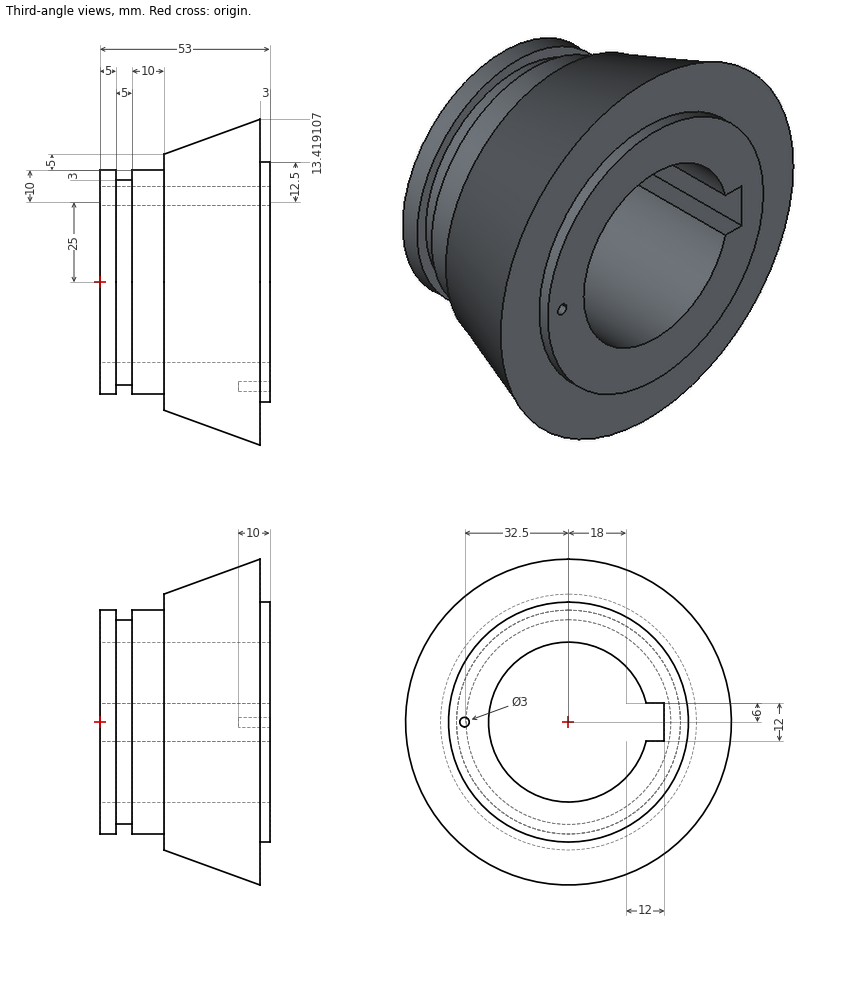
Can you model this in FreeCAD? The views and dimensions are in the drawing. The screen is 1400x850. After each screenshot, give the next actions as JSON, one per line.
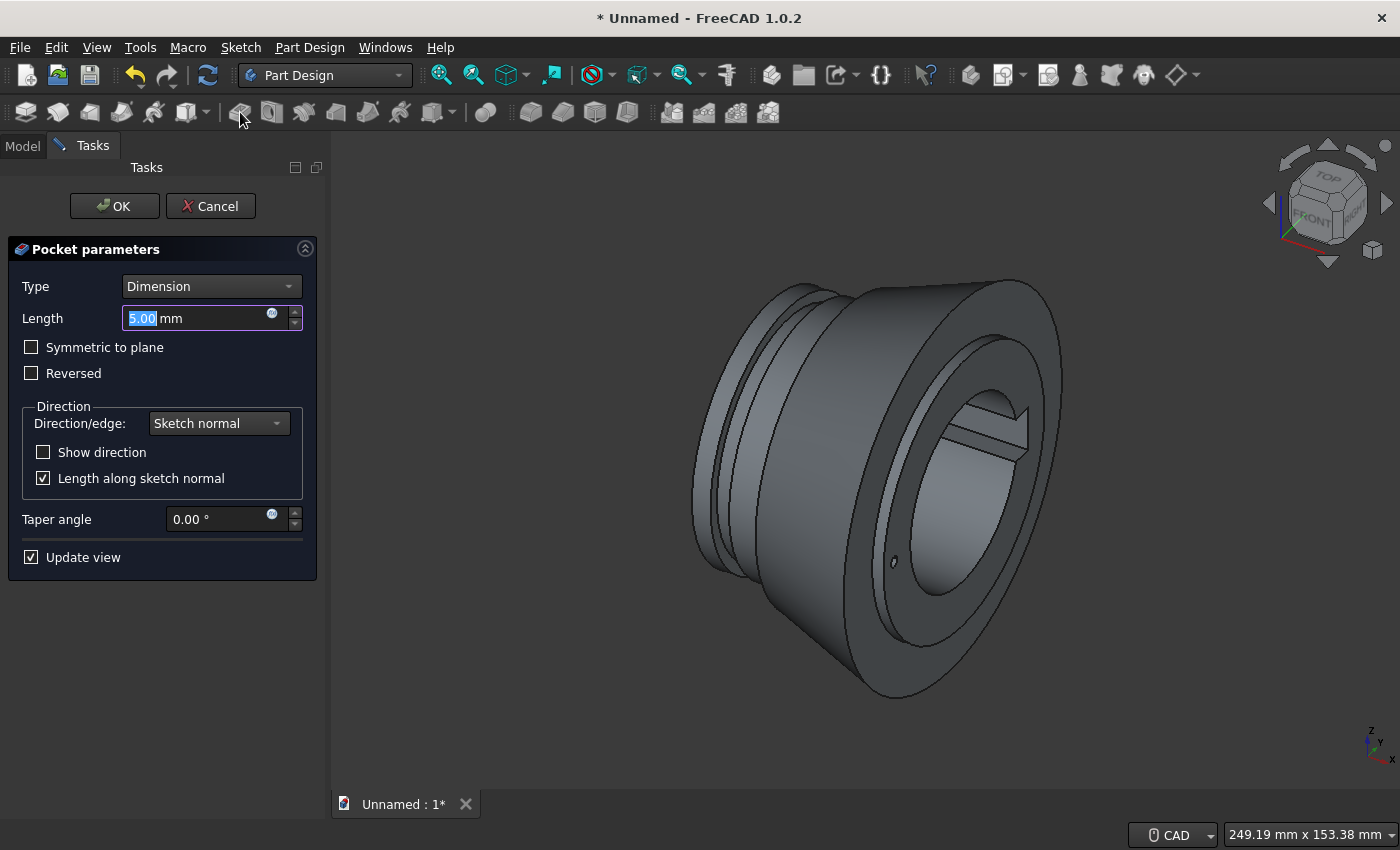
{"action": "type", "text": "10"}
{"action": "key", "text": "Tab"}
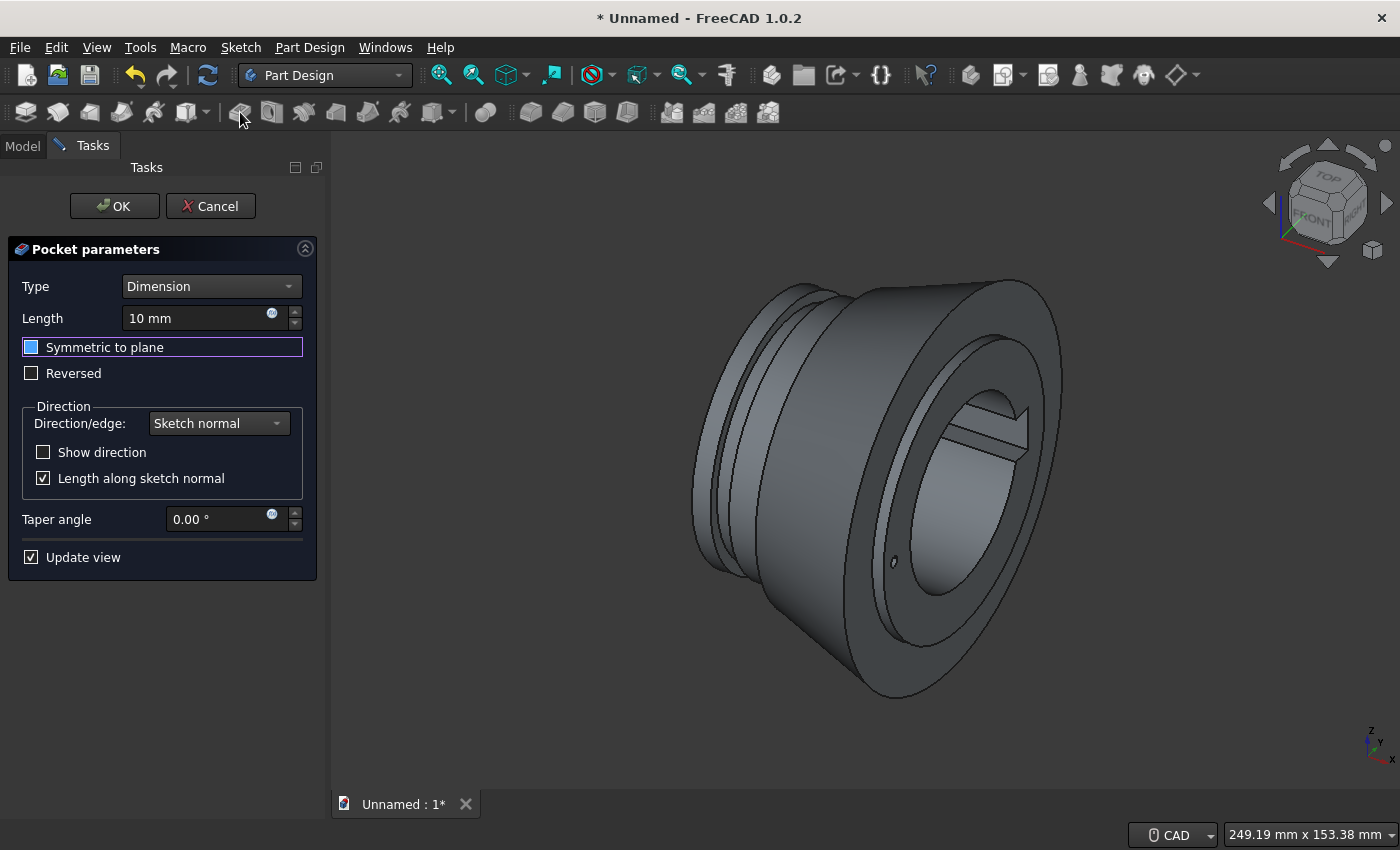
{"action": "left_click", "coordinate": [115, 206]}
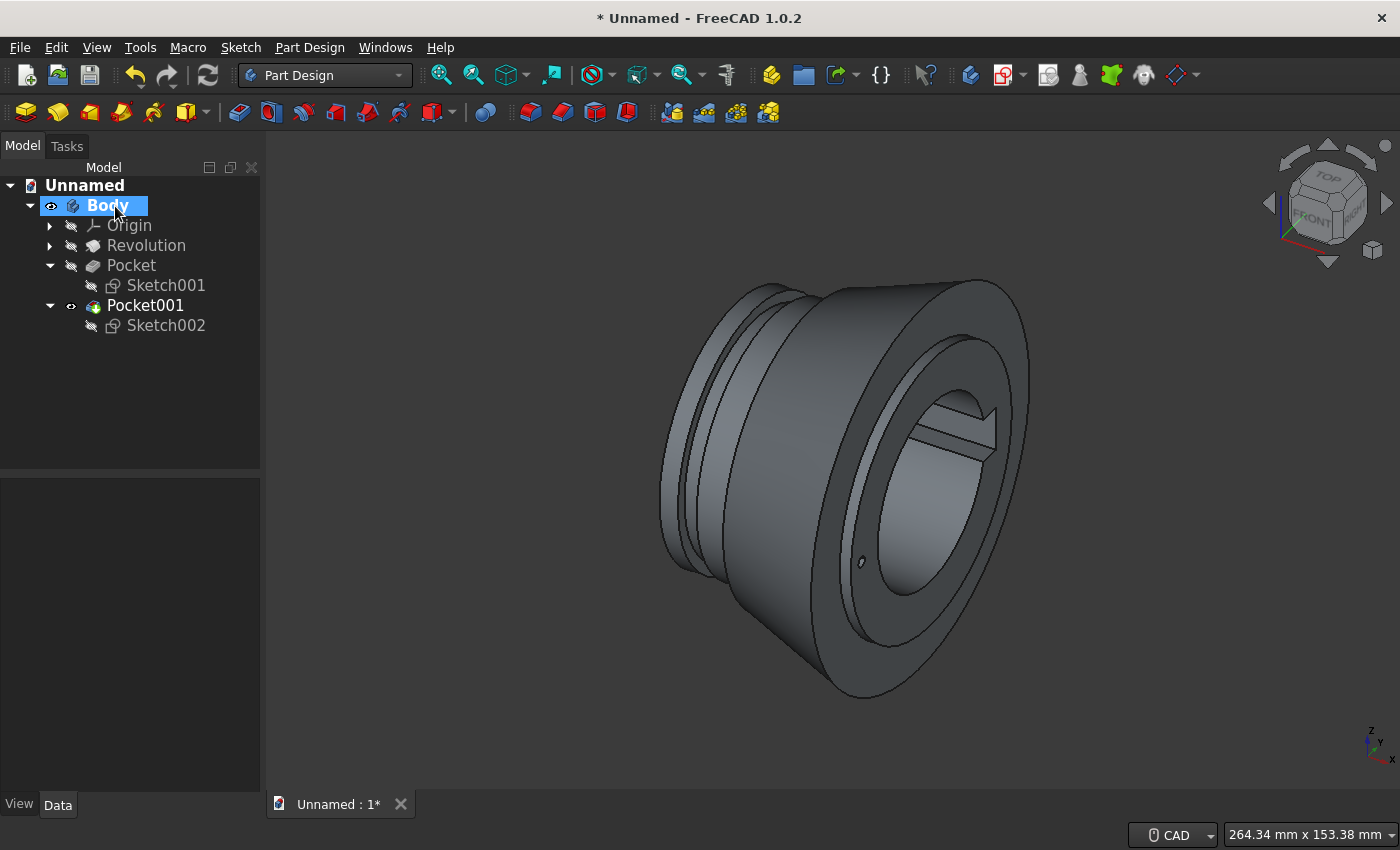
{"action": "key", "text": "0"}